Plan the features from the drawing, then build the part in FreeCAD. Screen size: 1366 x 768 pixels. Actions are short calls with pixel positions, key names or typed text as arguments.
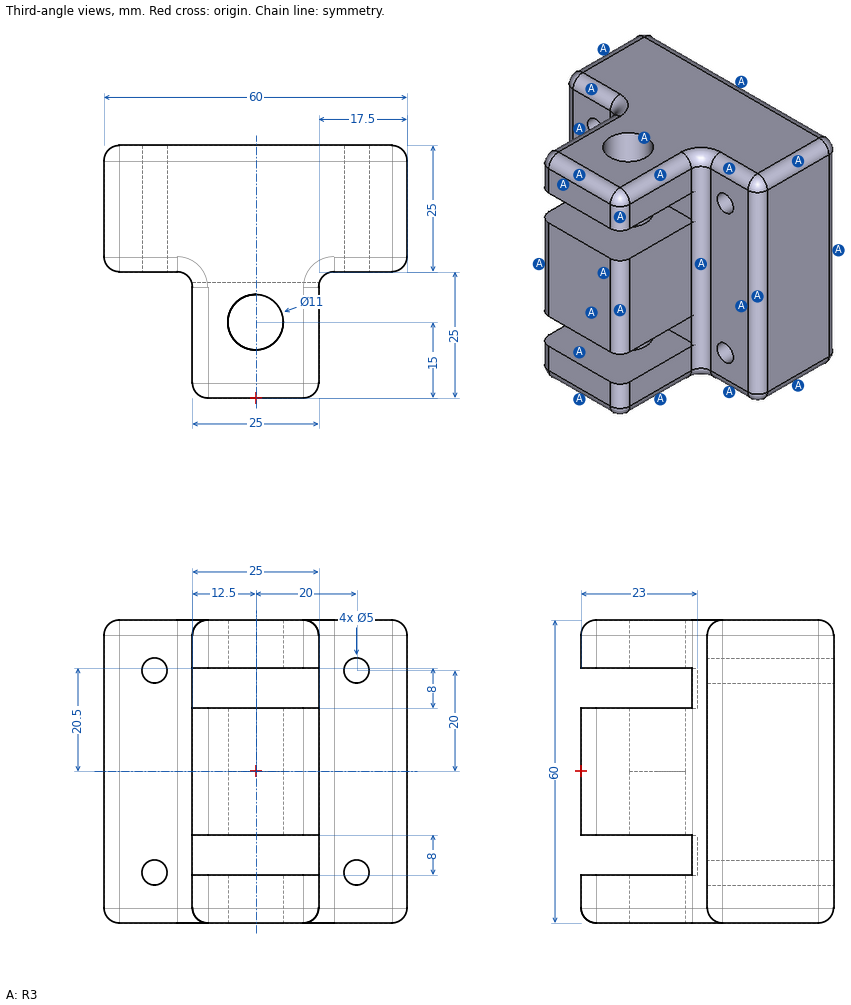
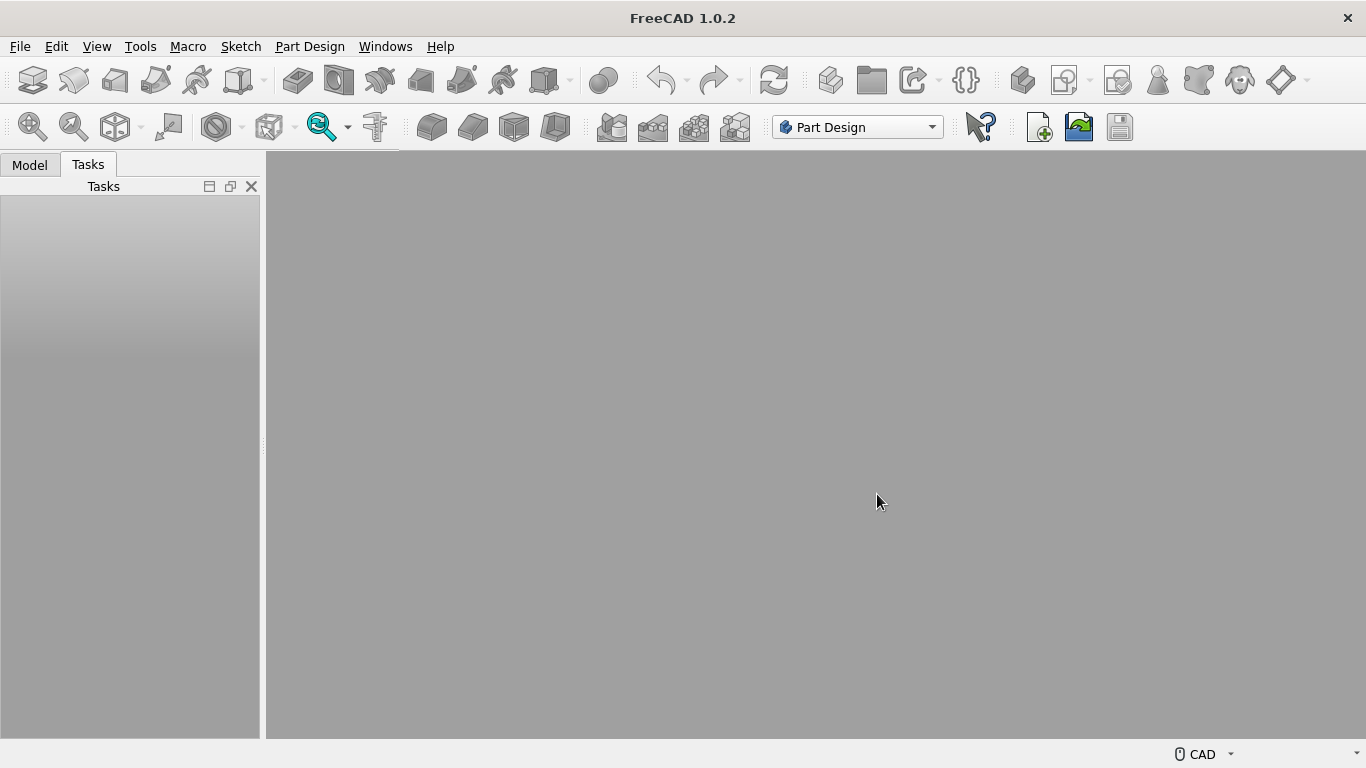
key(ctrl+n)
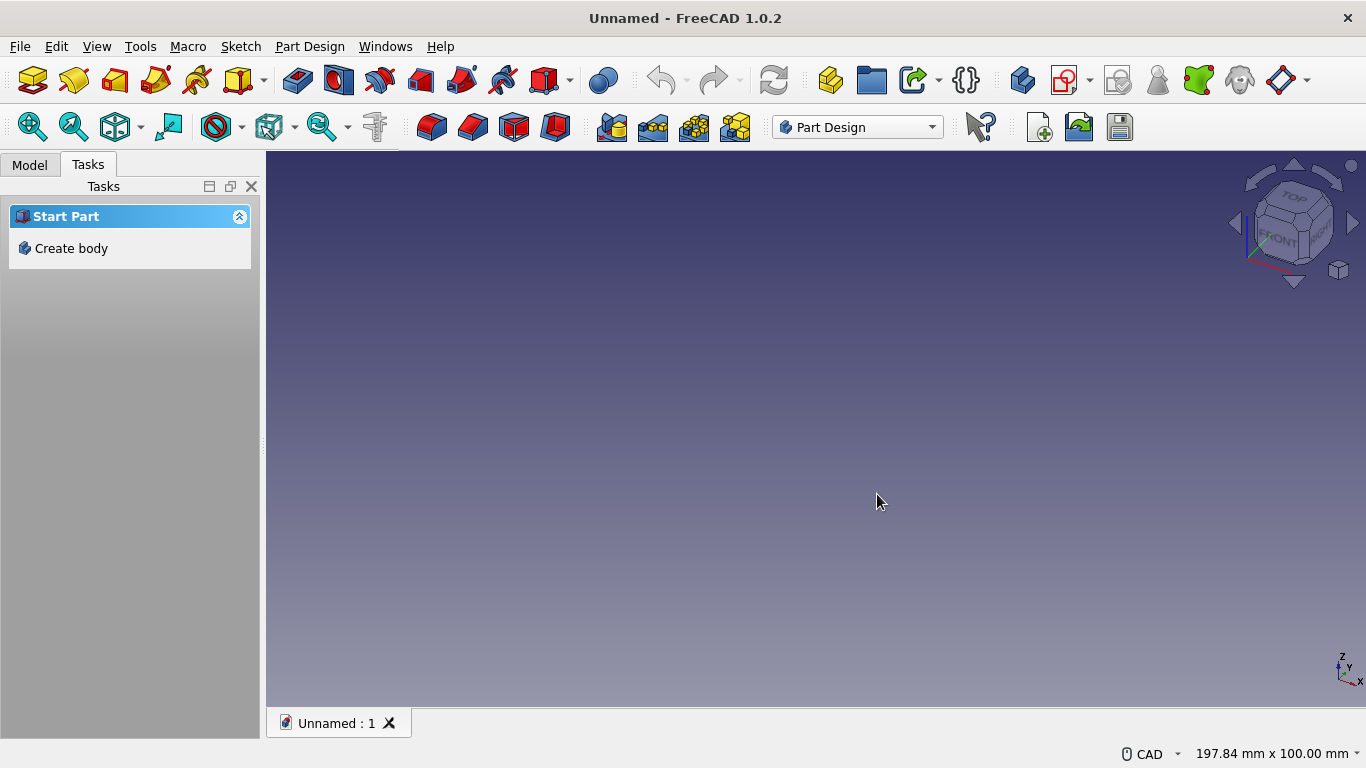
click(1064, 80)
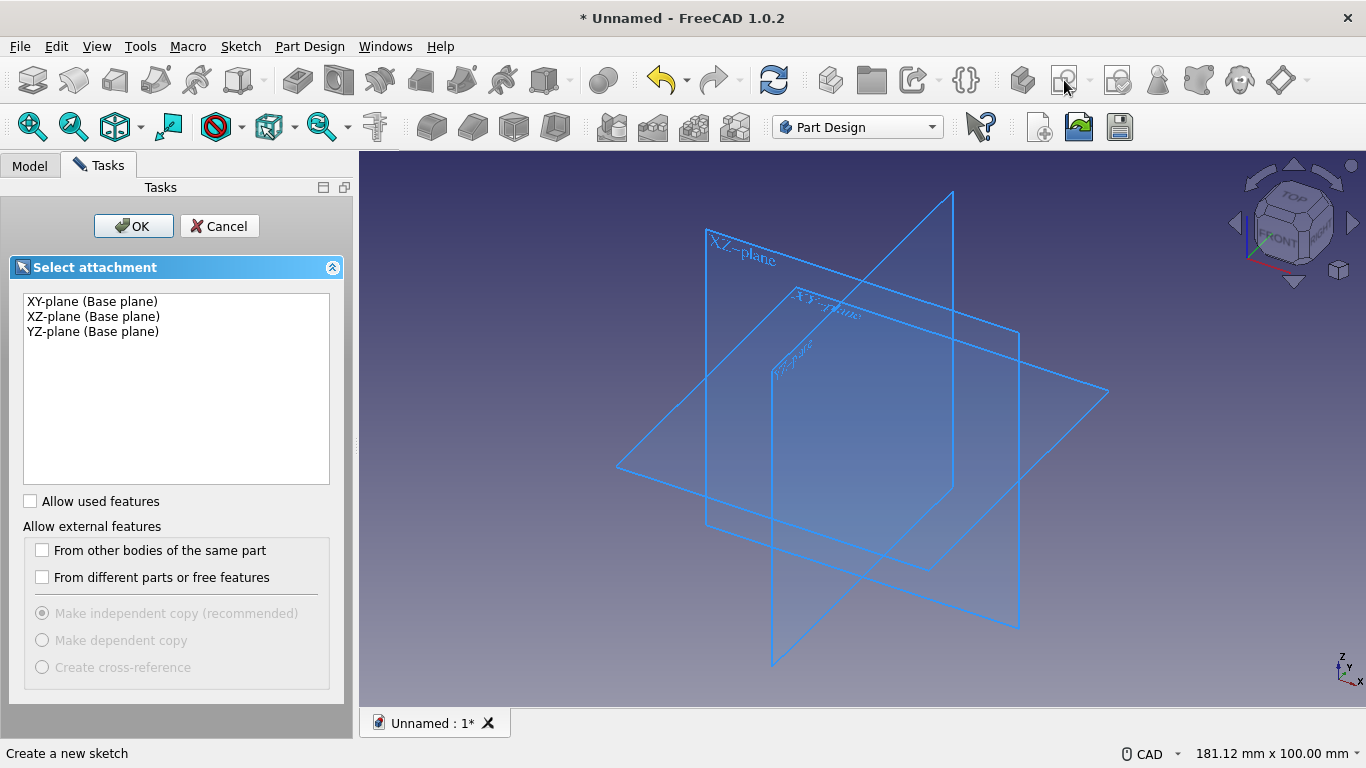
click(84, 302)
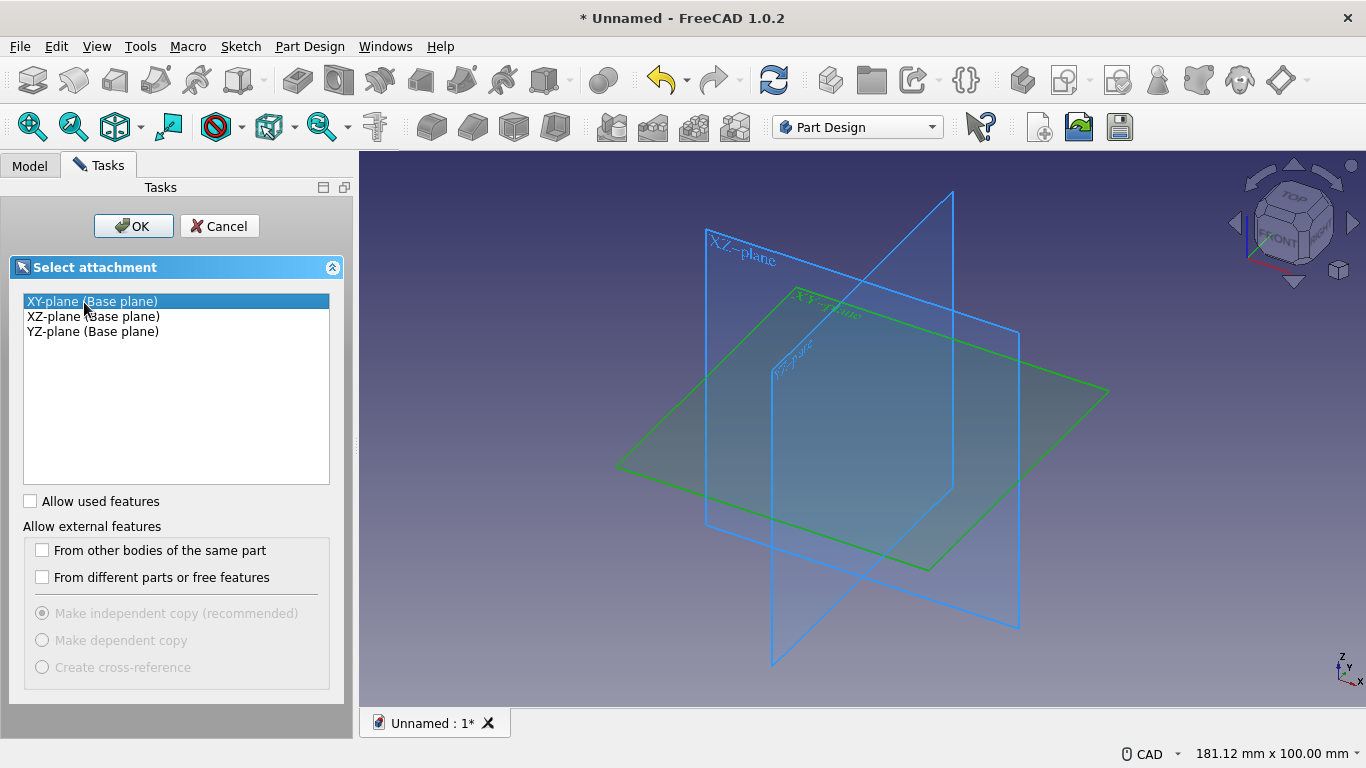
click(134, 226)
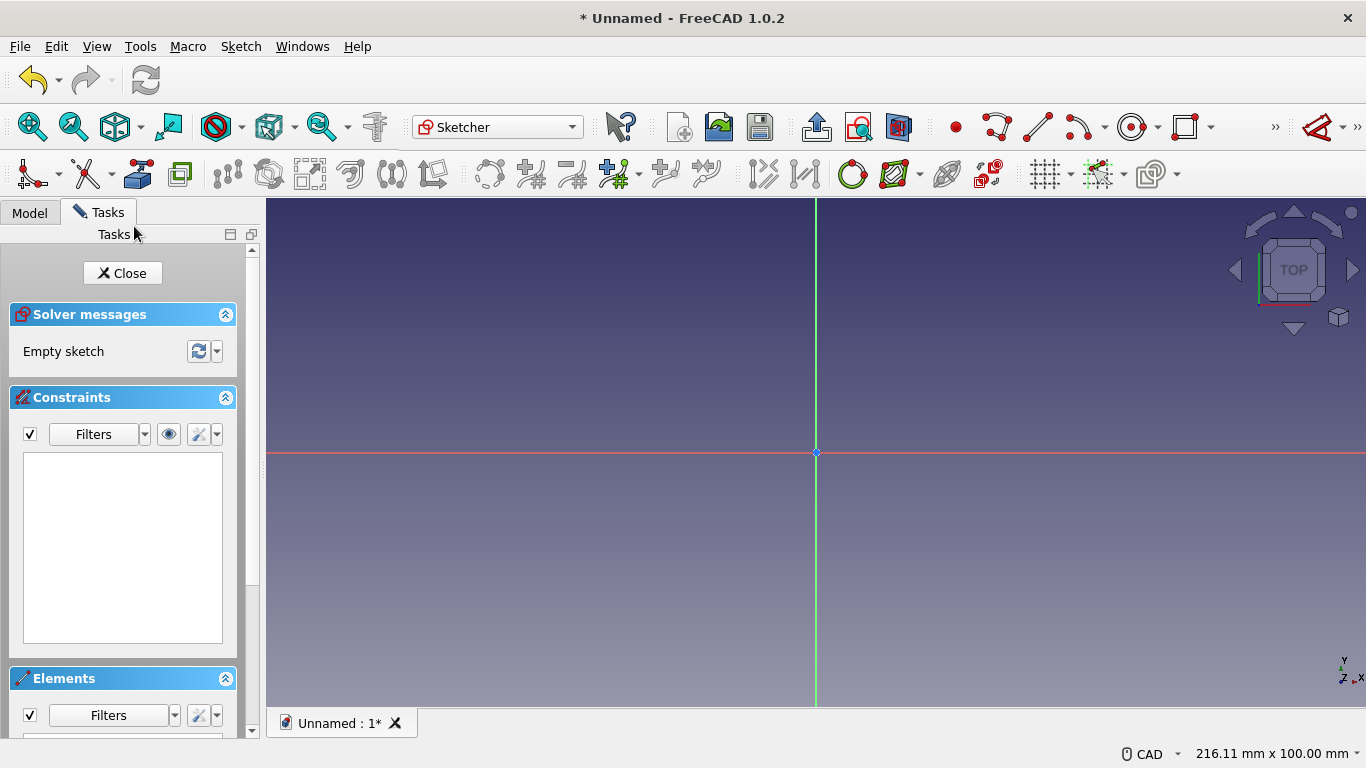
scroll(438, 679, down, 1)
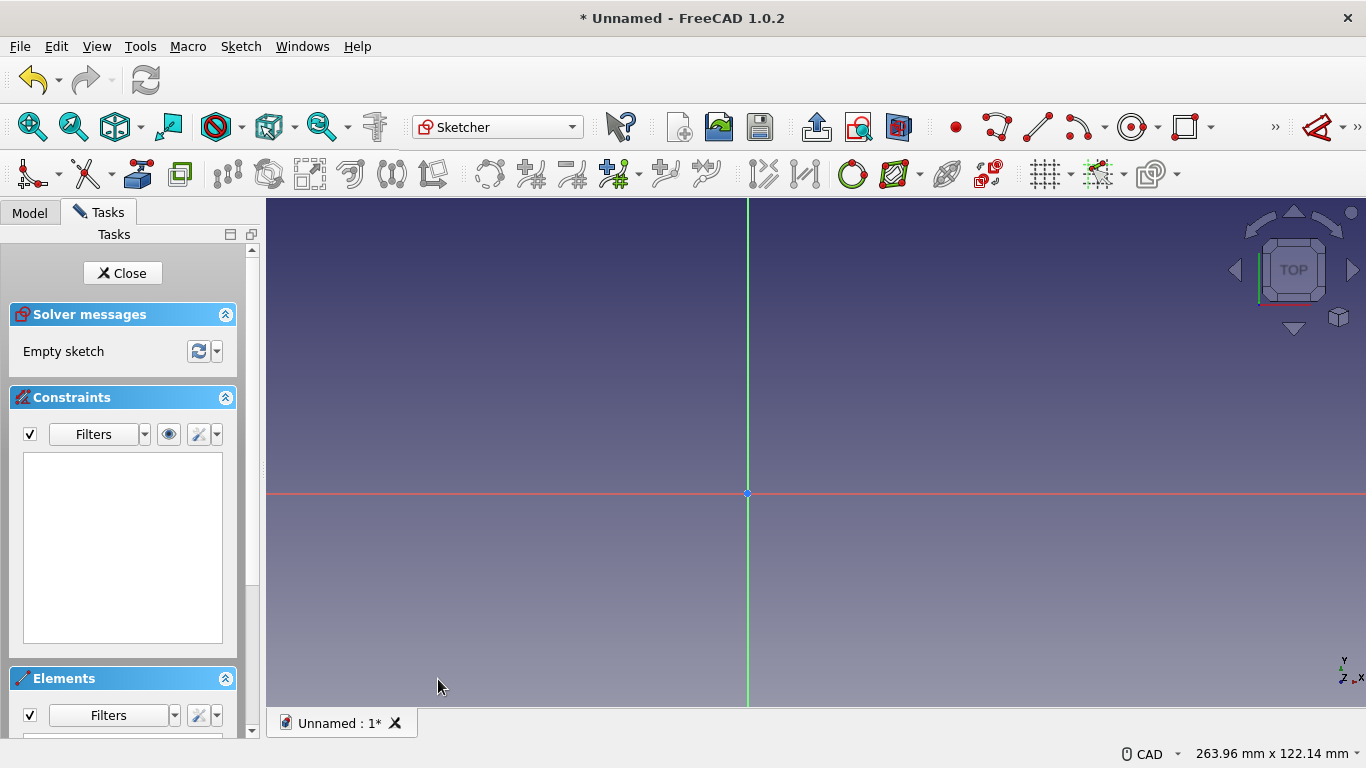
scroll(748, 262, up, 2)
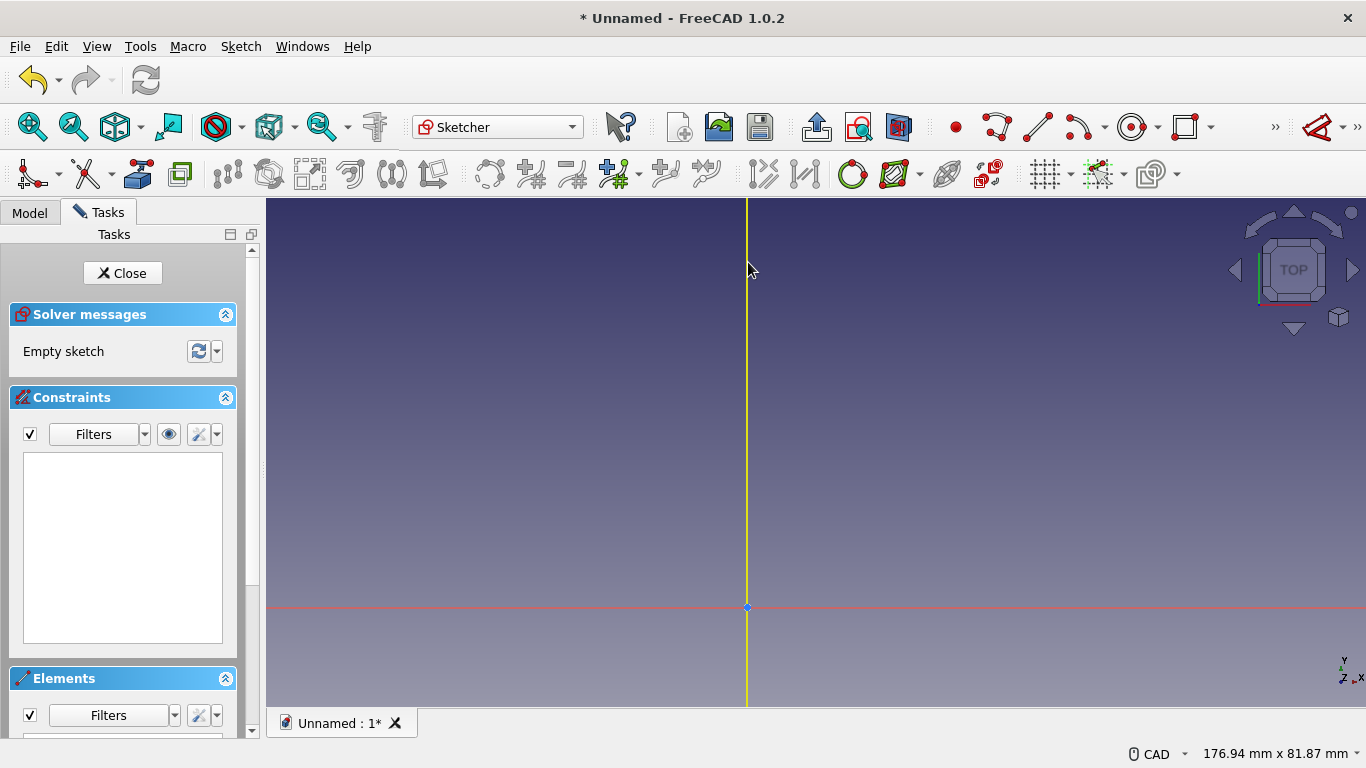
click(997, 128)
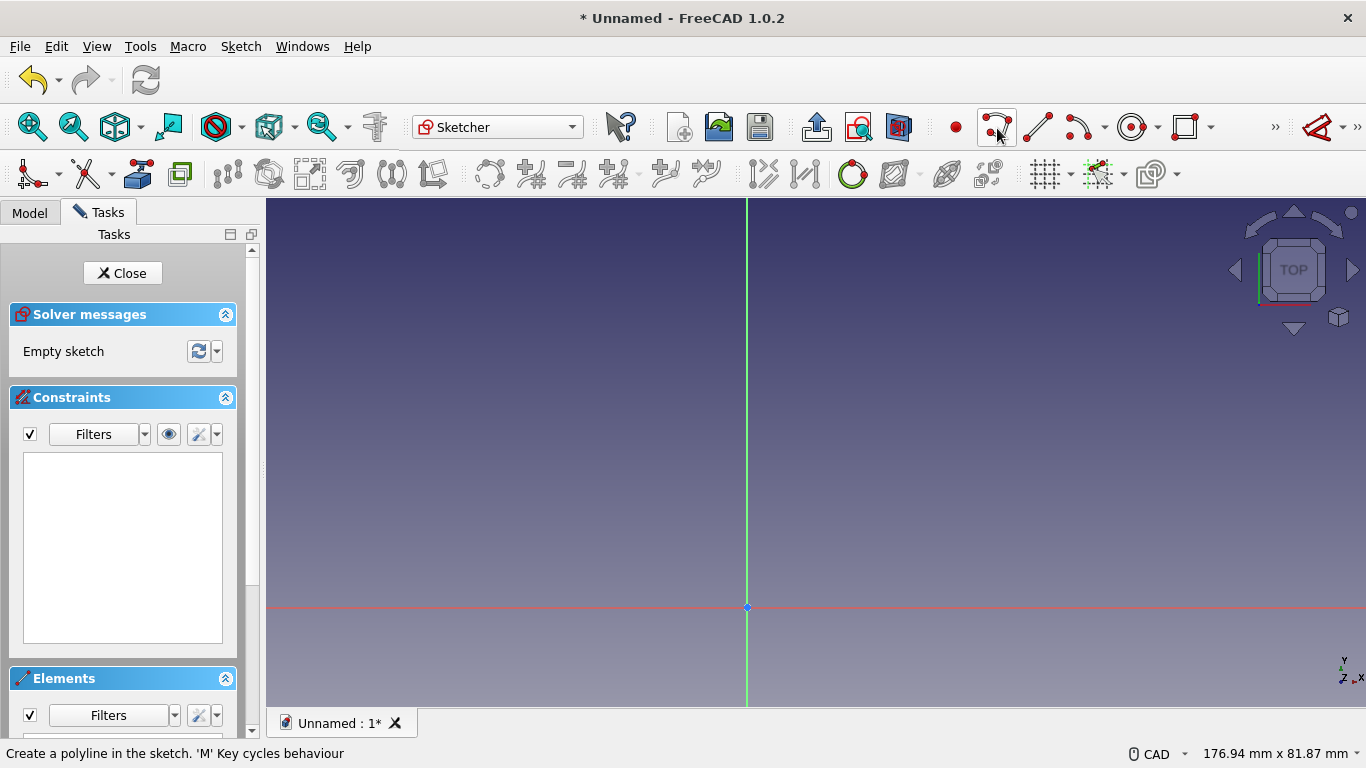
click(669, 608)
click(825, 599)
click(825, 452)
click(934, 452)
click(934, 297)
click(561, 297)
click(561, 452)
click(669, 452)
click(669, 608)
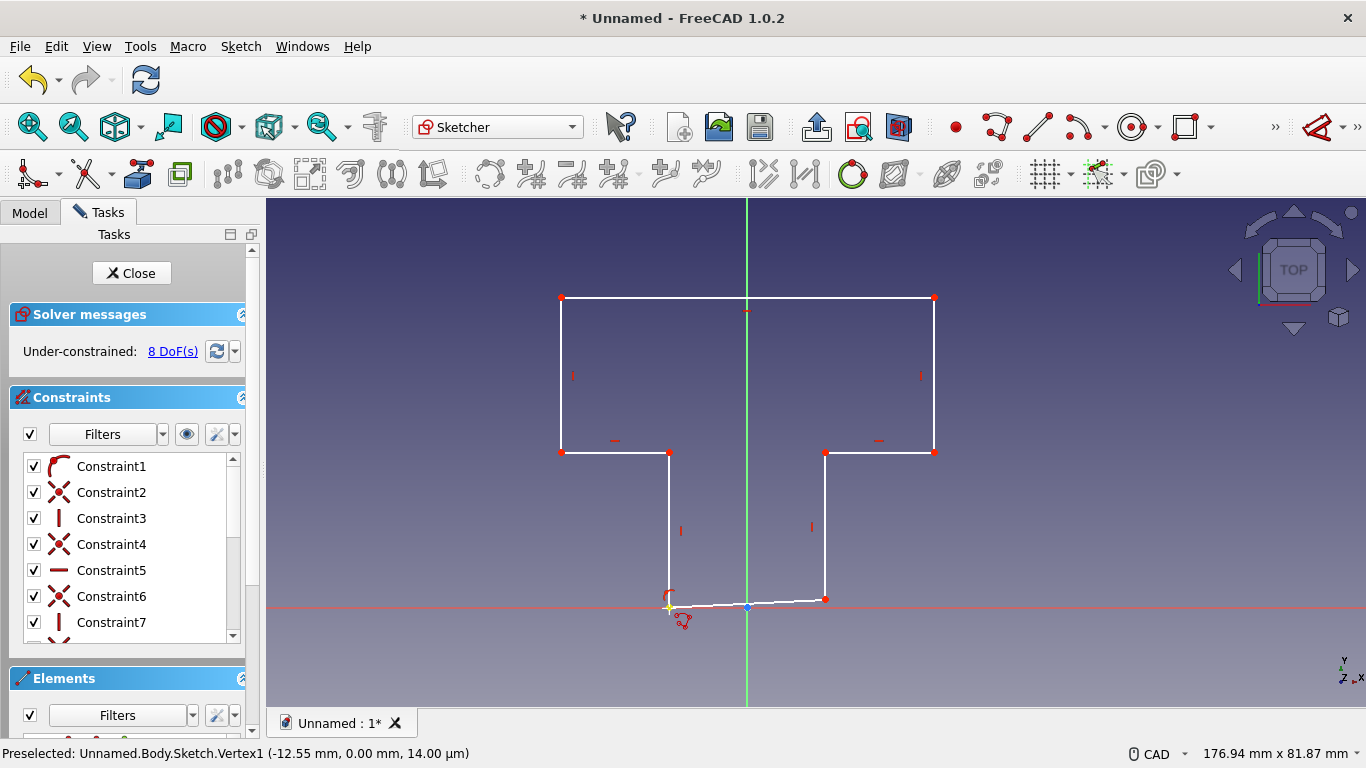
click(1132, 128)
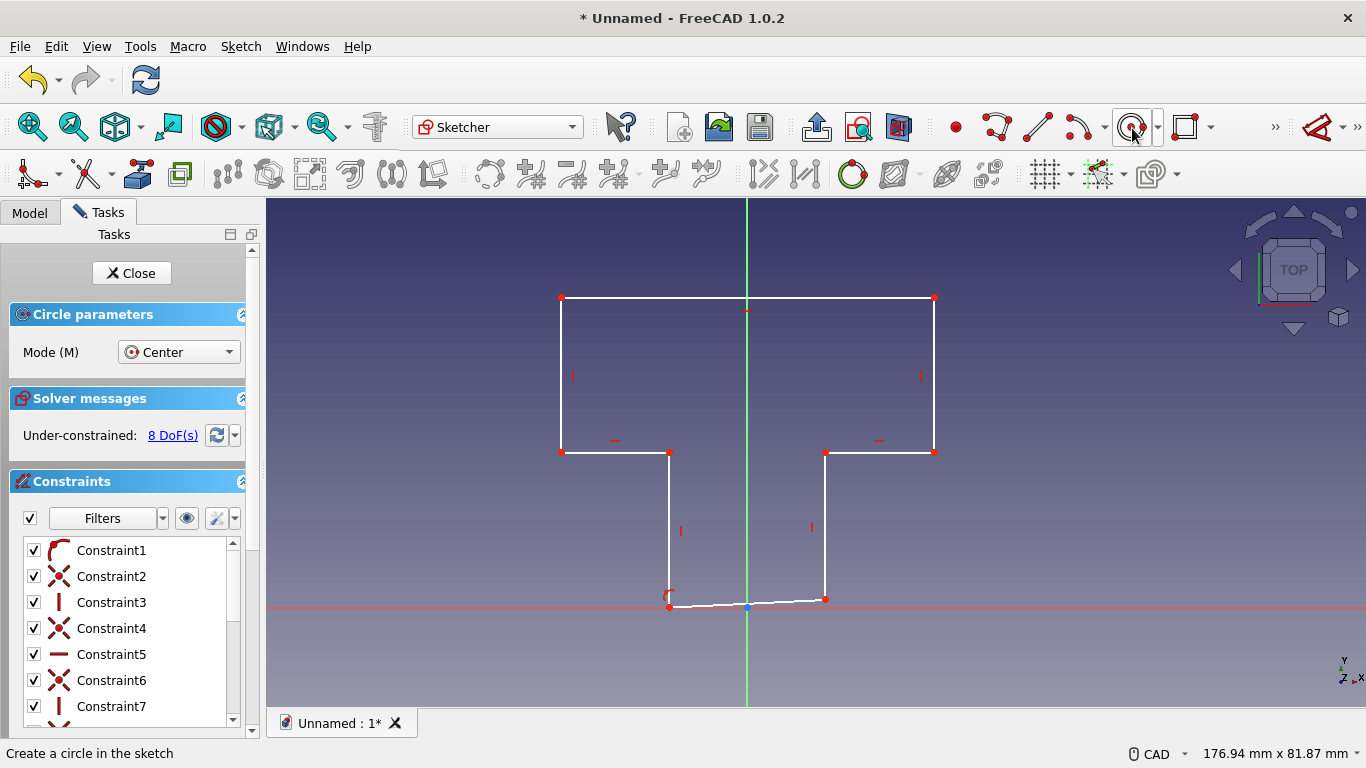
click(747, 514)
move(771, 490)